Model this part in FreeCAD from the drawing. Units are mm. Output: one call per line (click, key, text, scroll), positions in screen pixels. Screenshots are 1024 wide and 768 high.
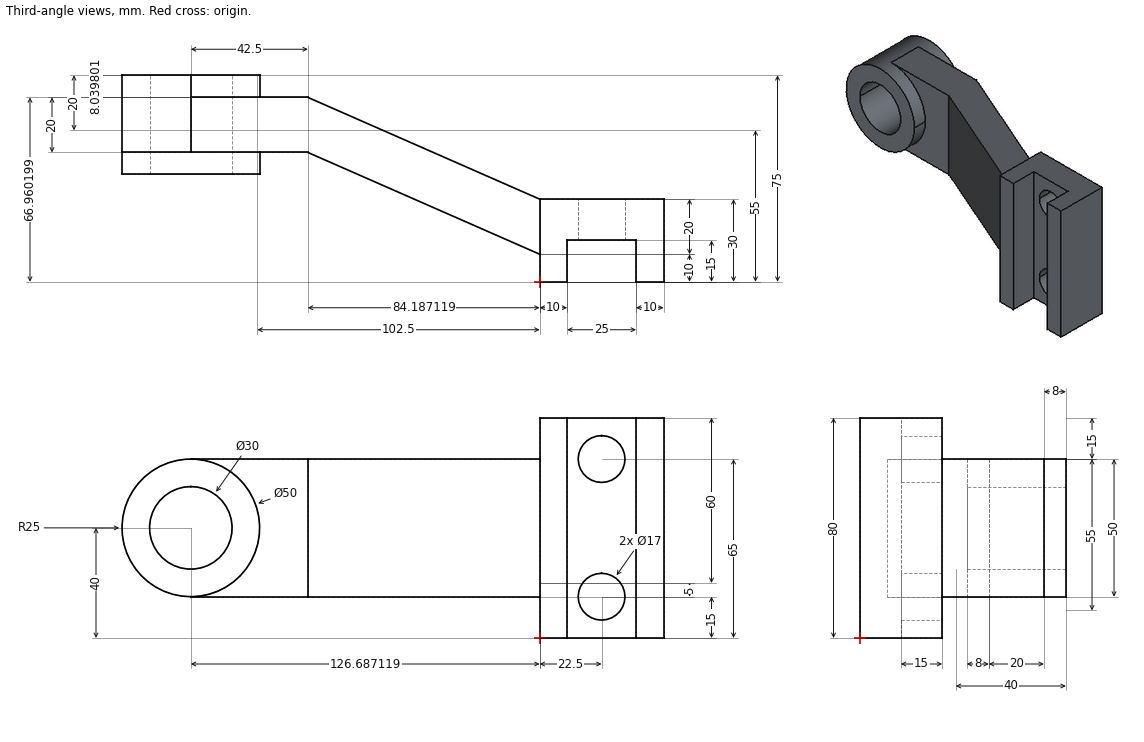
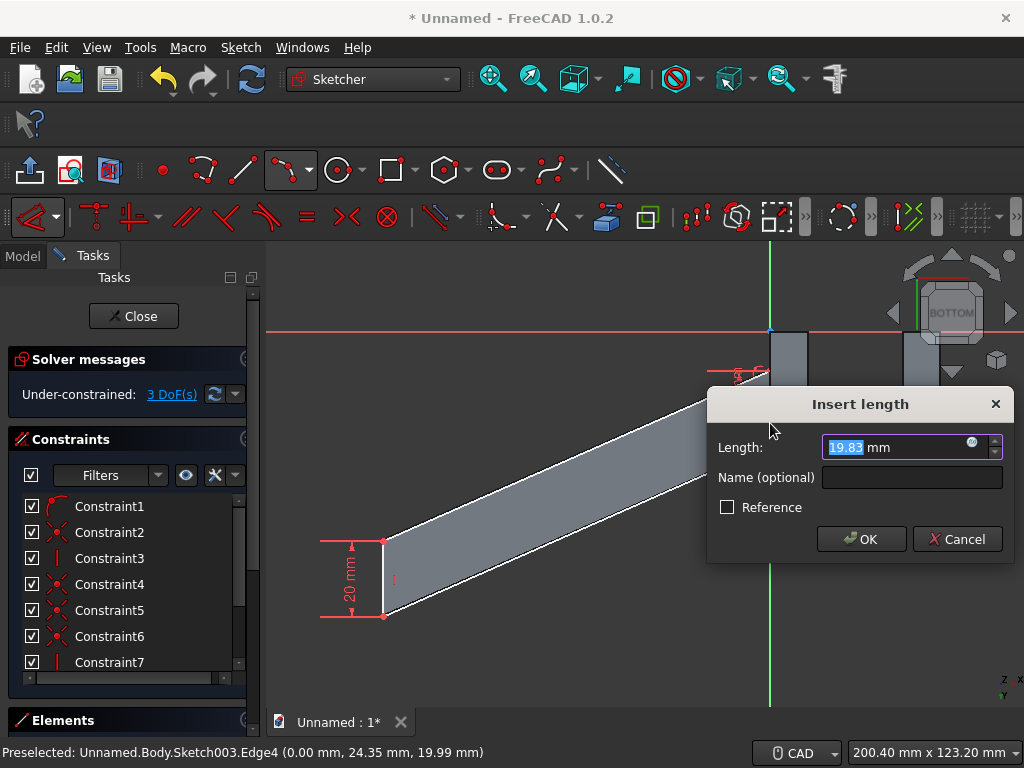
text(20)
key(Return)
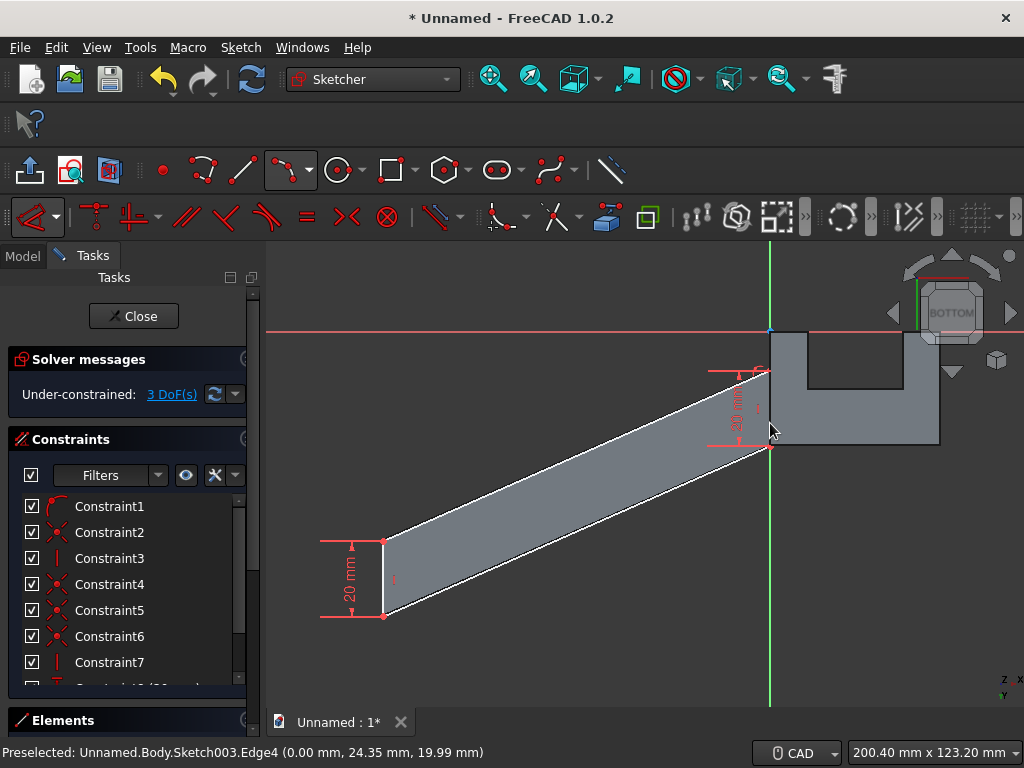
click(770, 371)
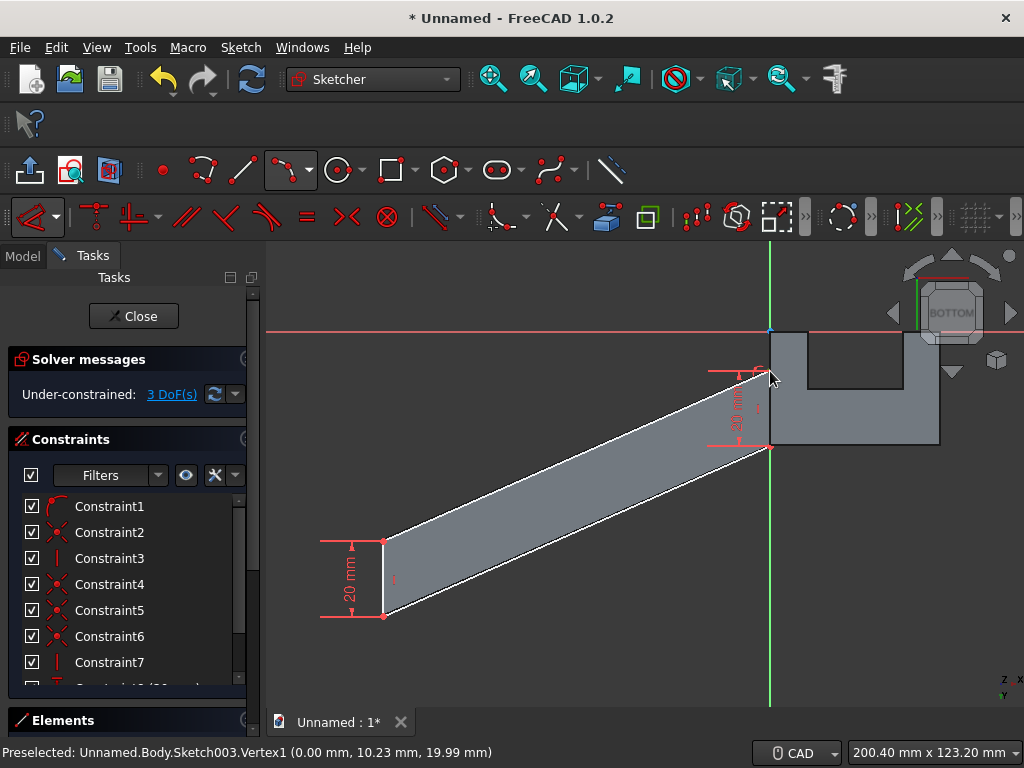
key(i)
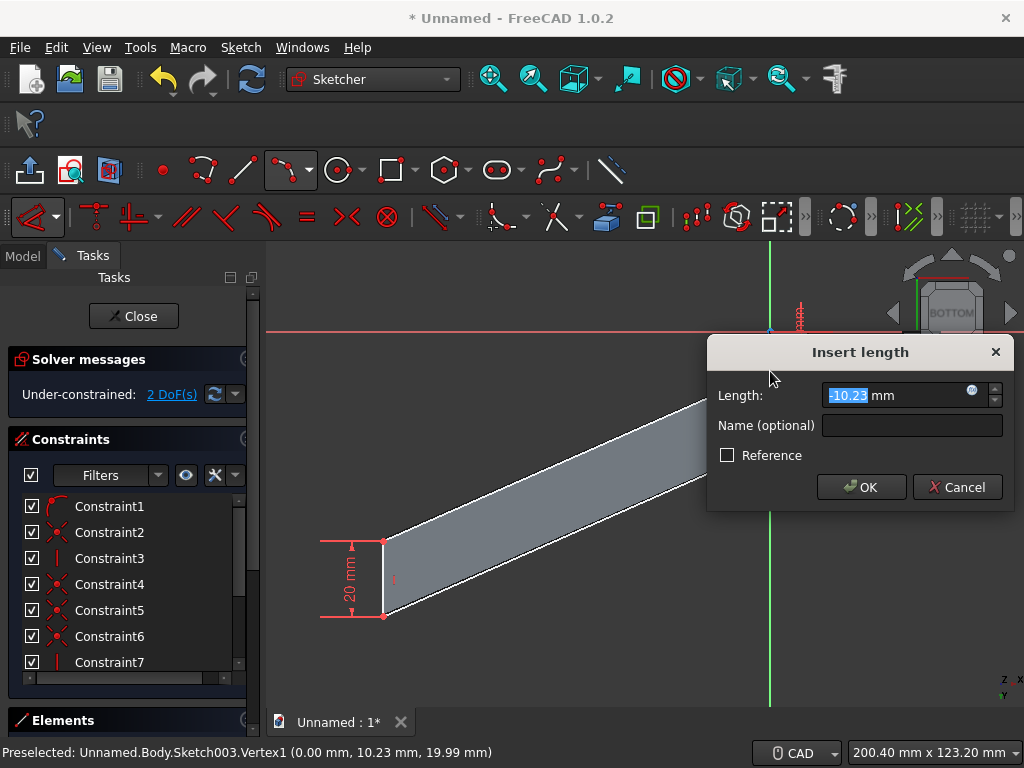
text(-10)
key(Return)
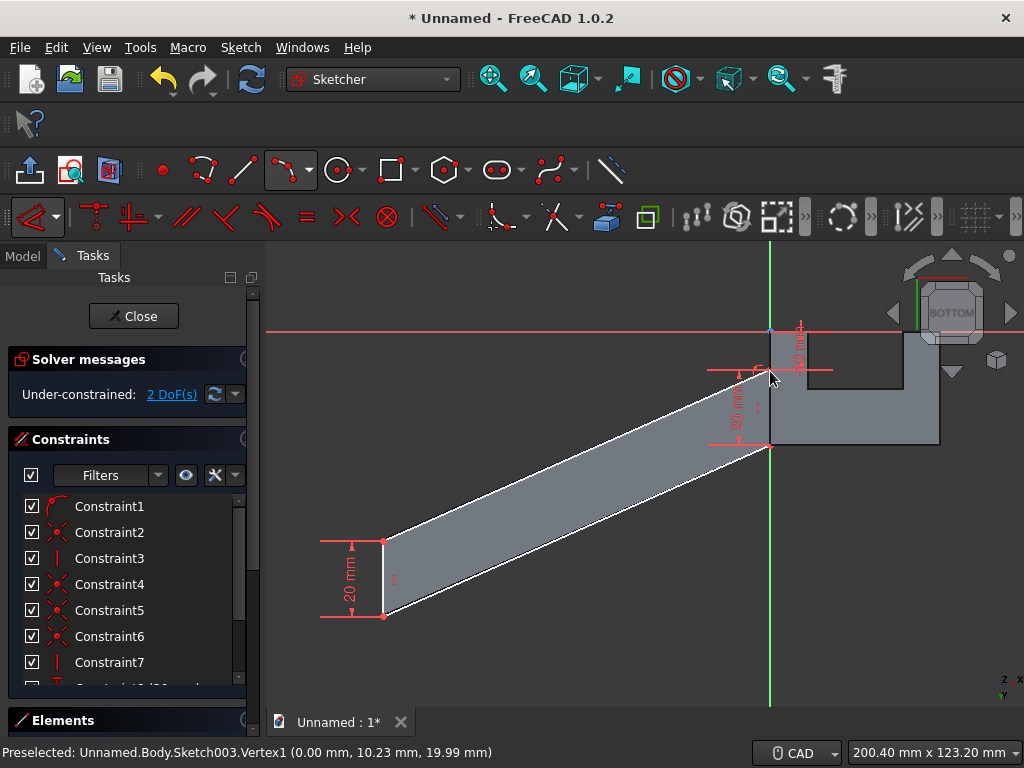
click(383, 541)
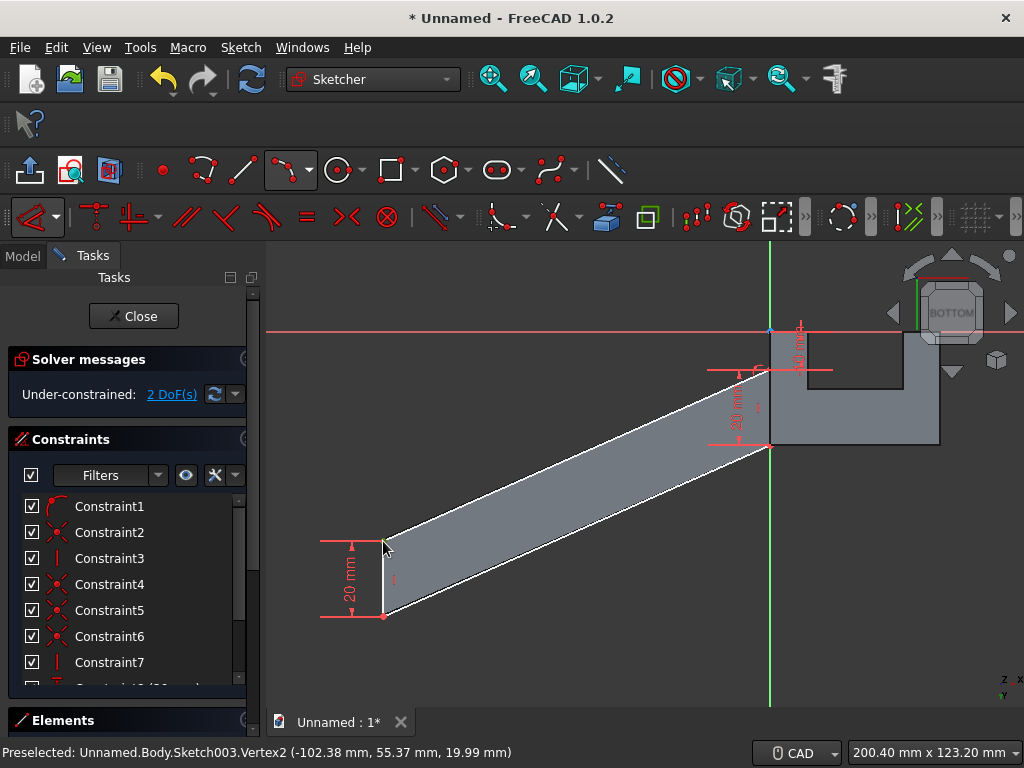
click(58, 218)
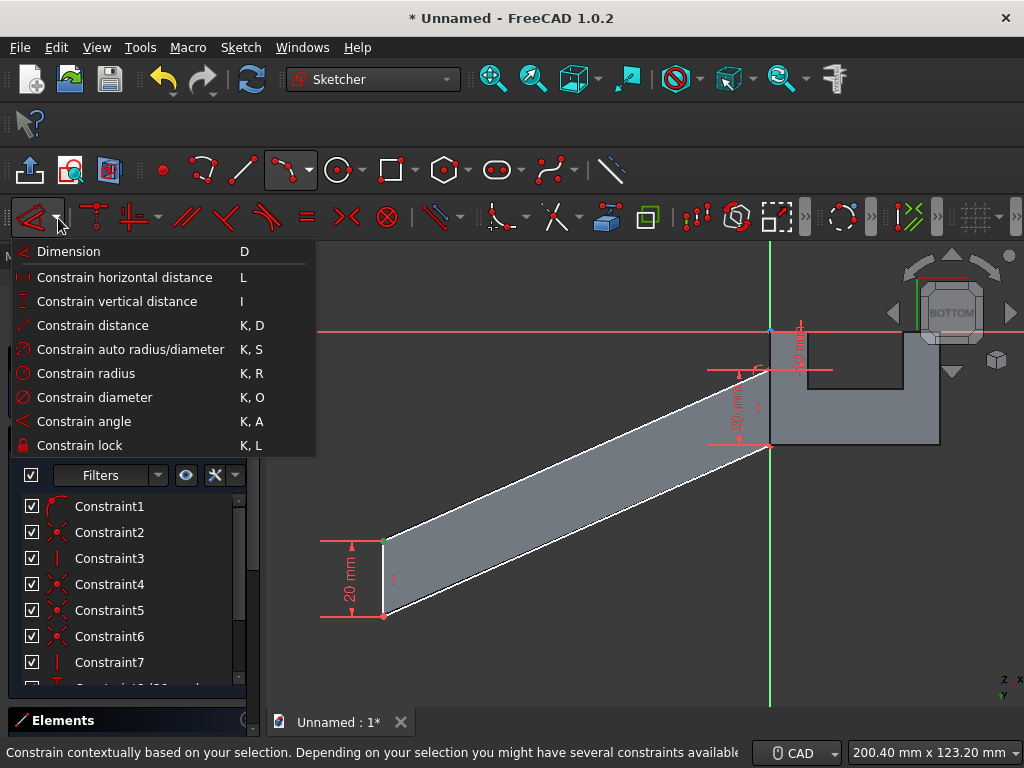
click(164, 301)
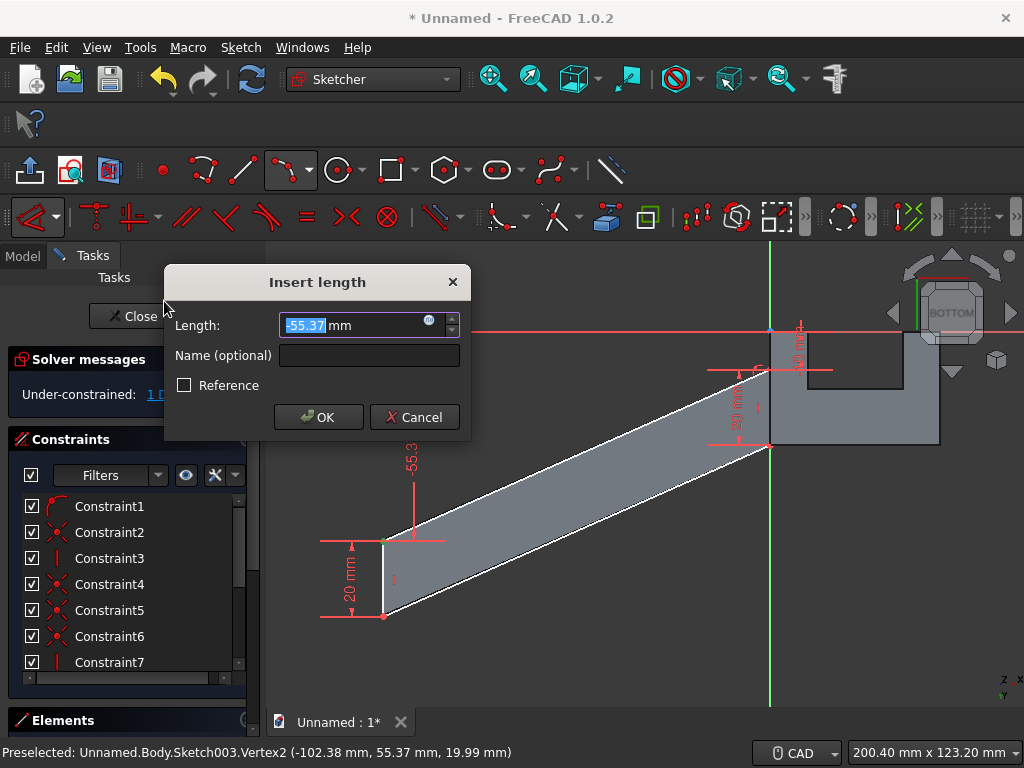
text(-55)
key(Return)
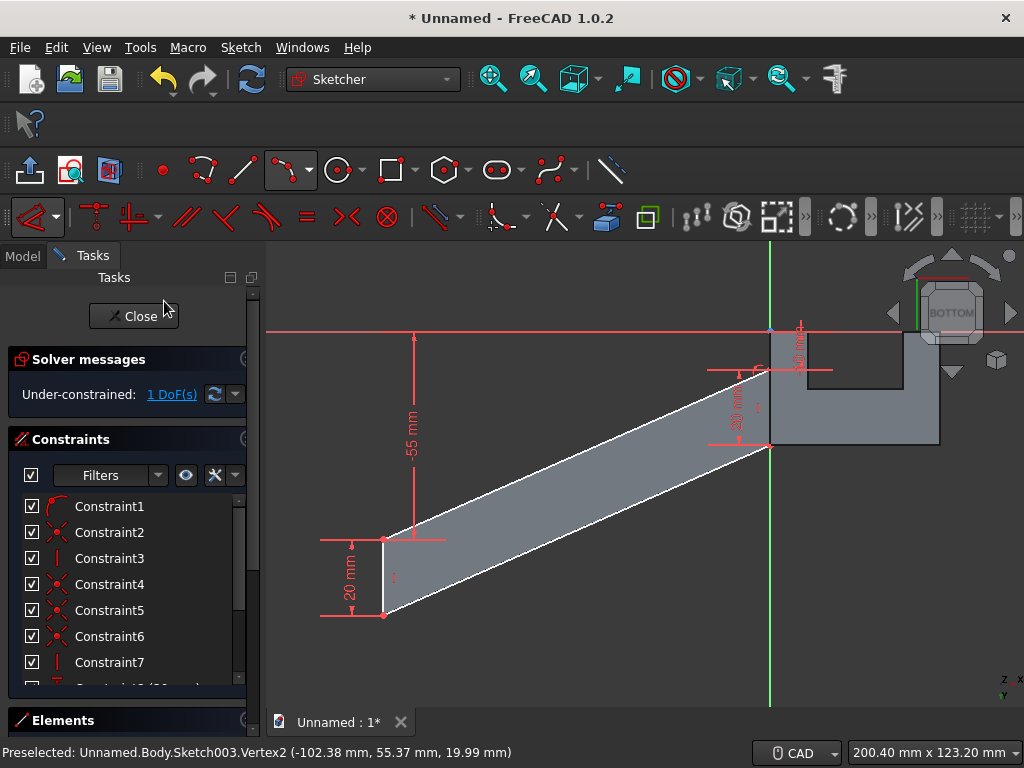
click(383, 540)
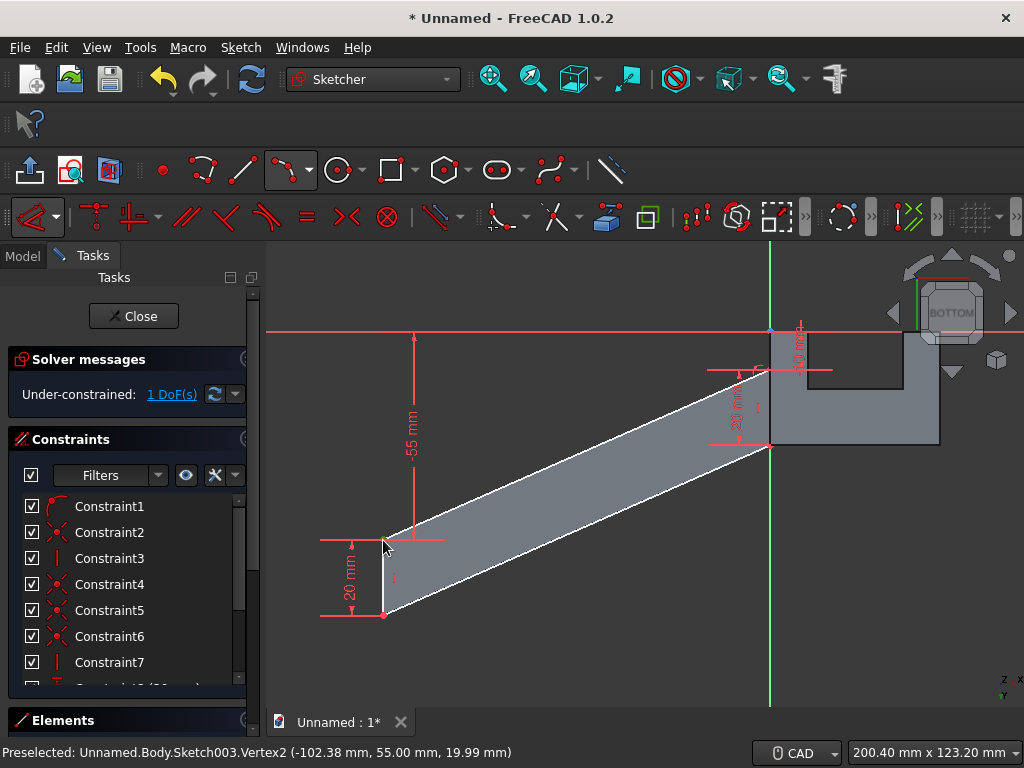
key(l)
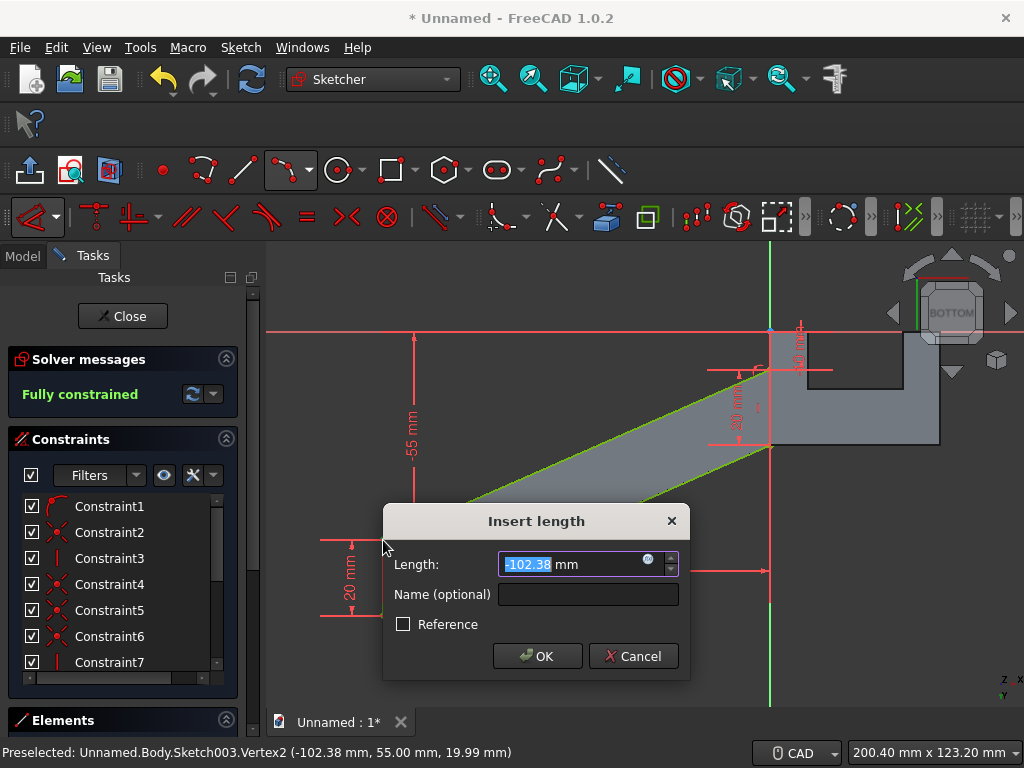
text(-102.5)
key(Return)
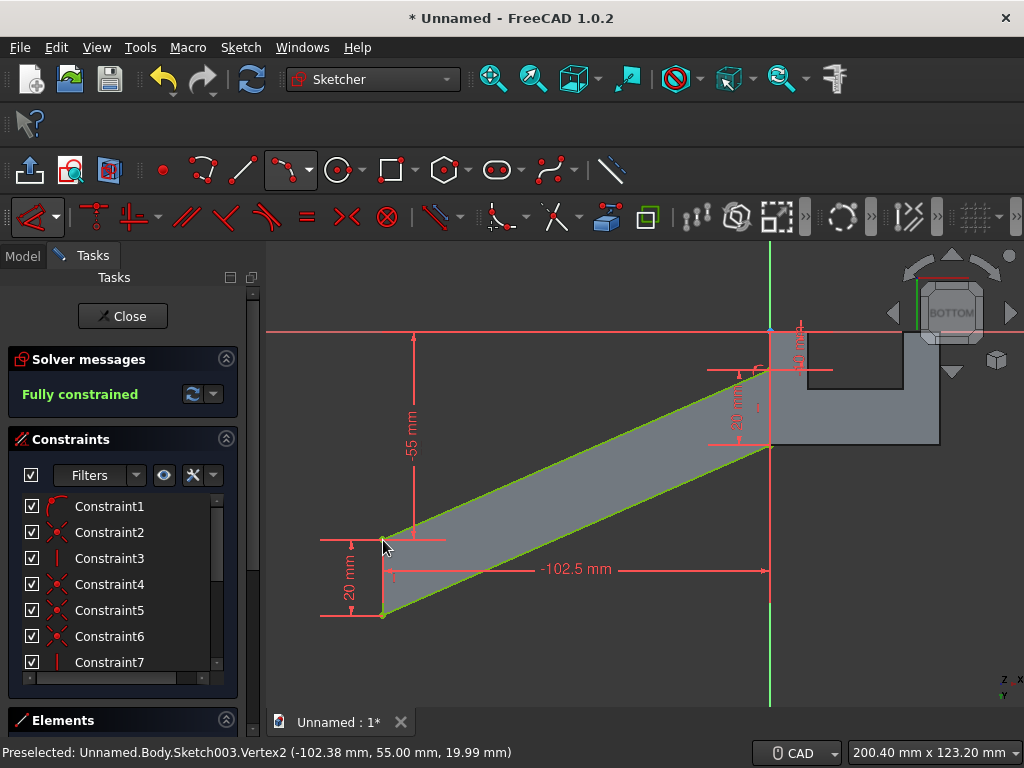
click(123, 316)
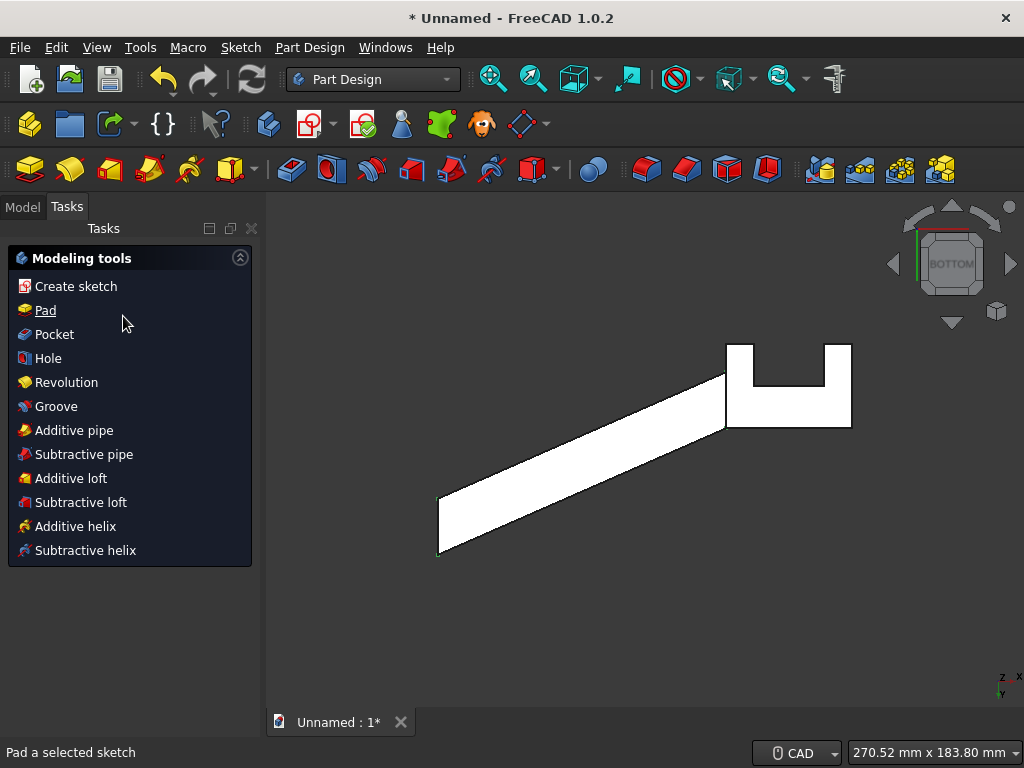
click(30, 170)